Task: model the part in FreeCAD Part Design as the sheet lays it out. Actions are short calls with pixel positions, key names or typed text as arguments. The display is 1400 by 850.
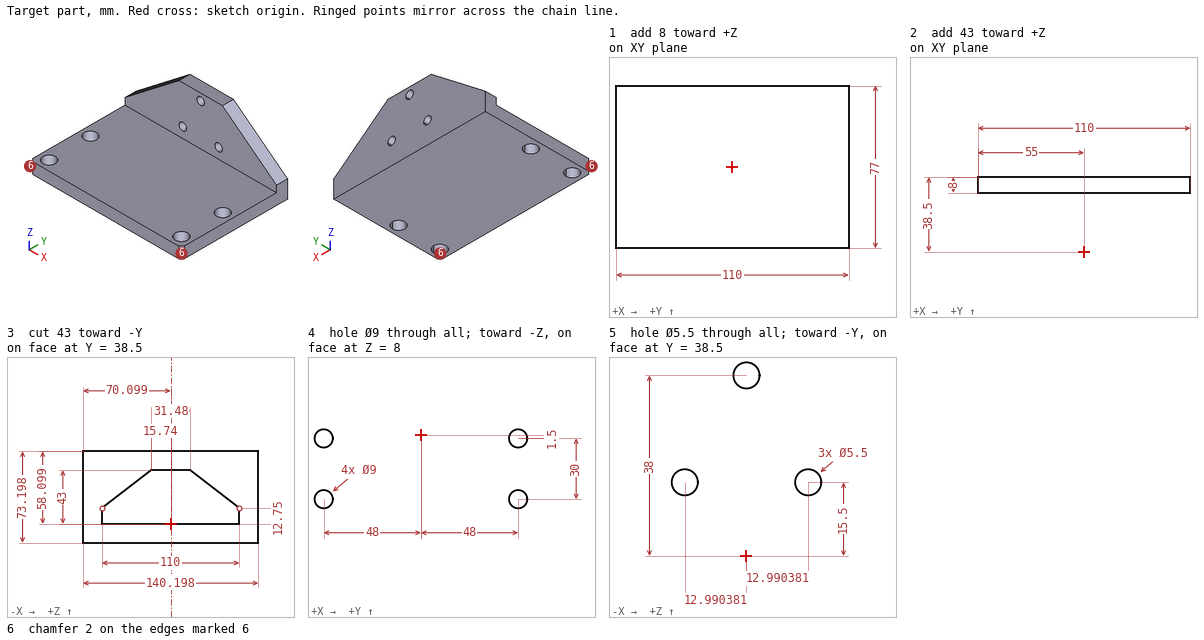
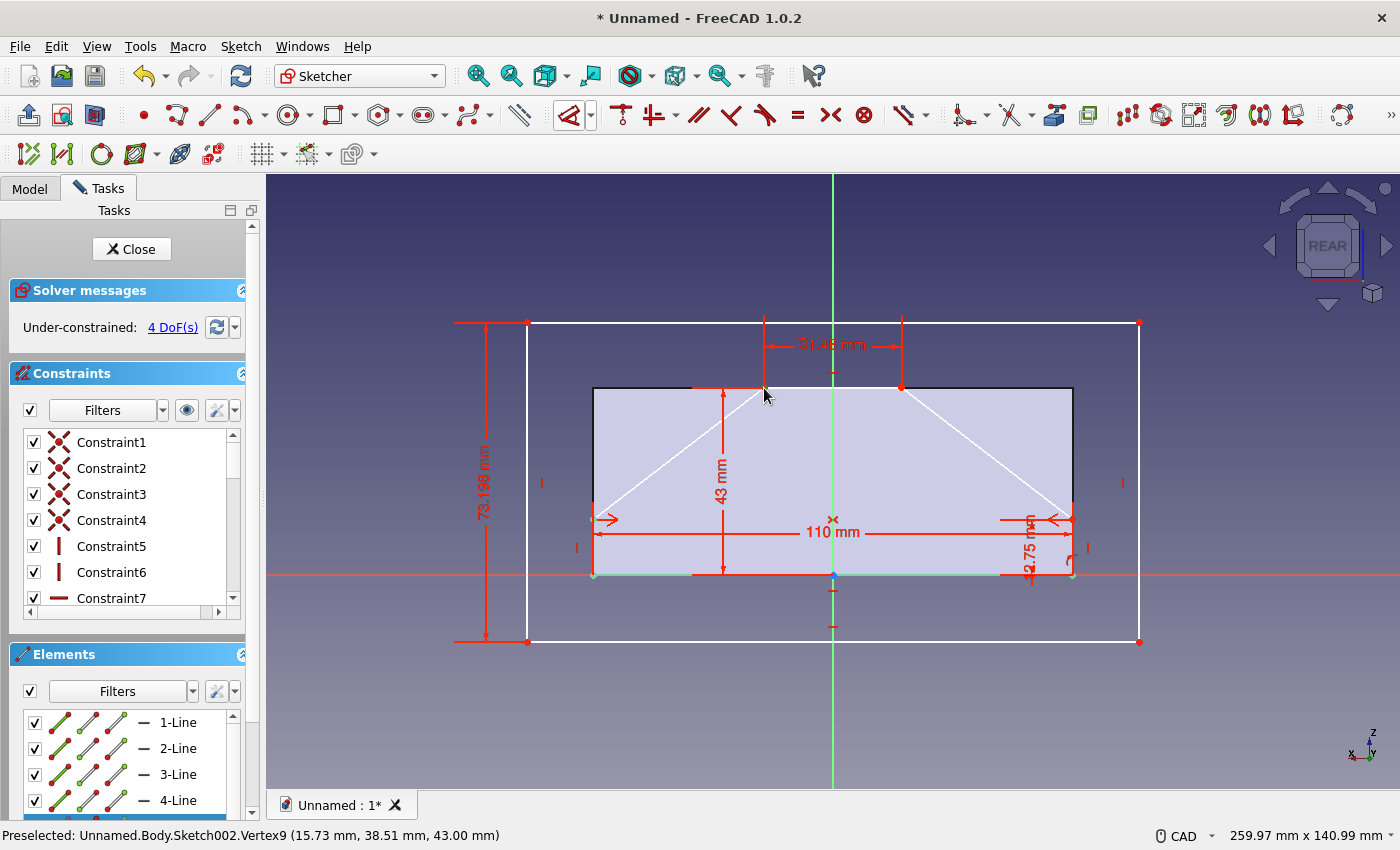
key(l)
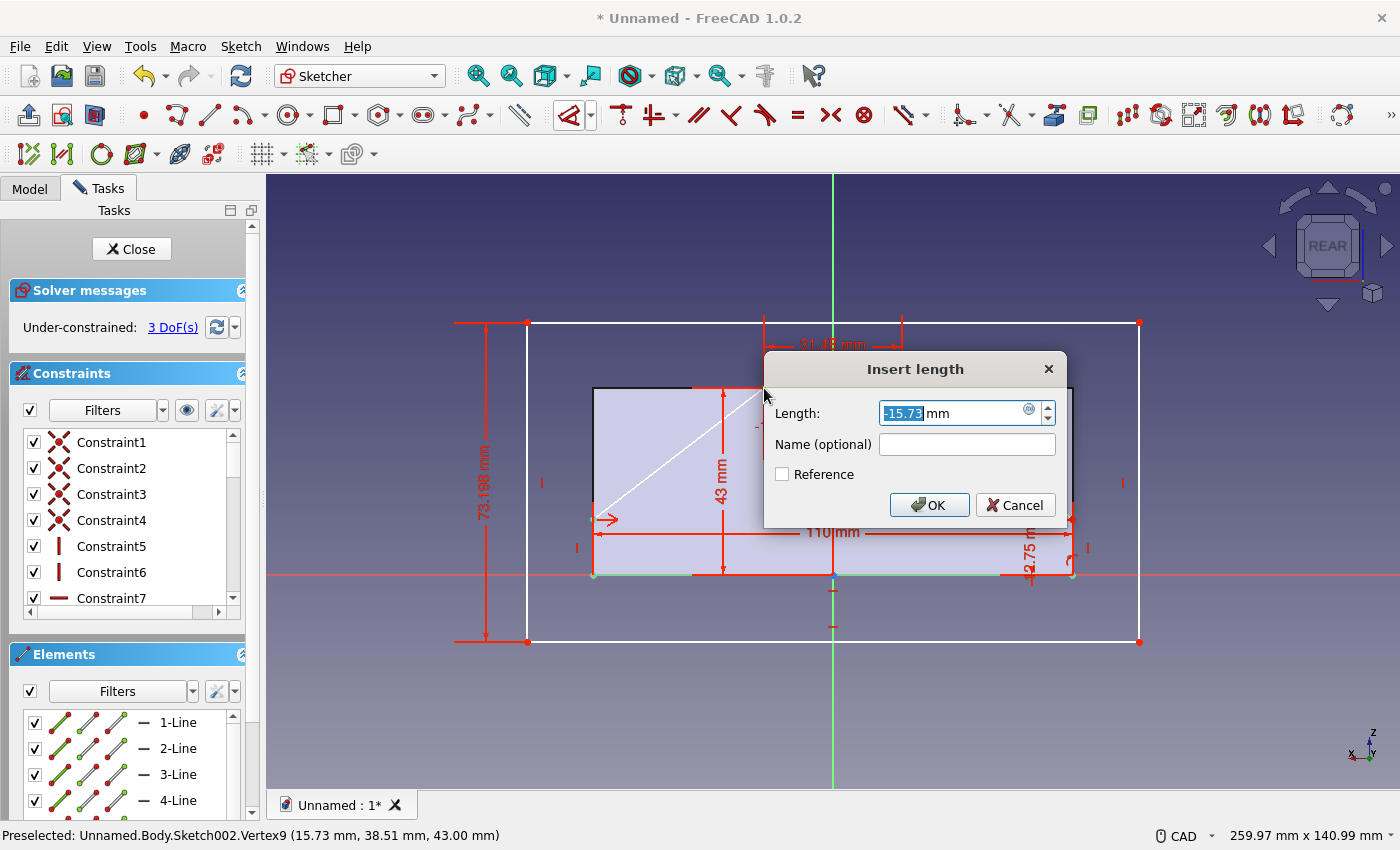
text(-15.74)
key(Return)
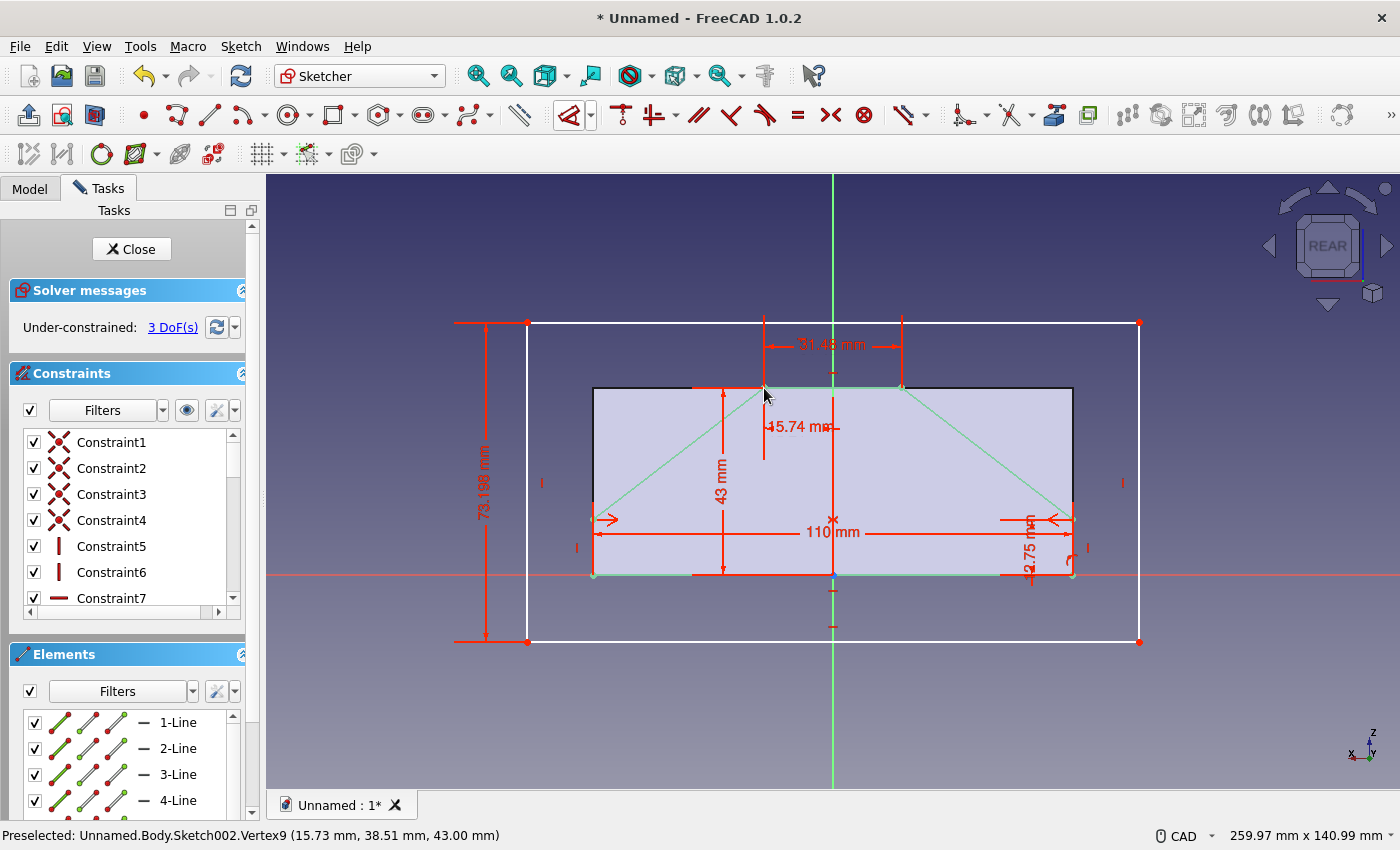
click(711, 642)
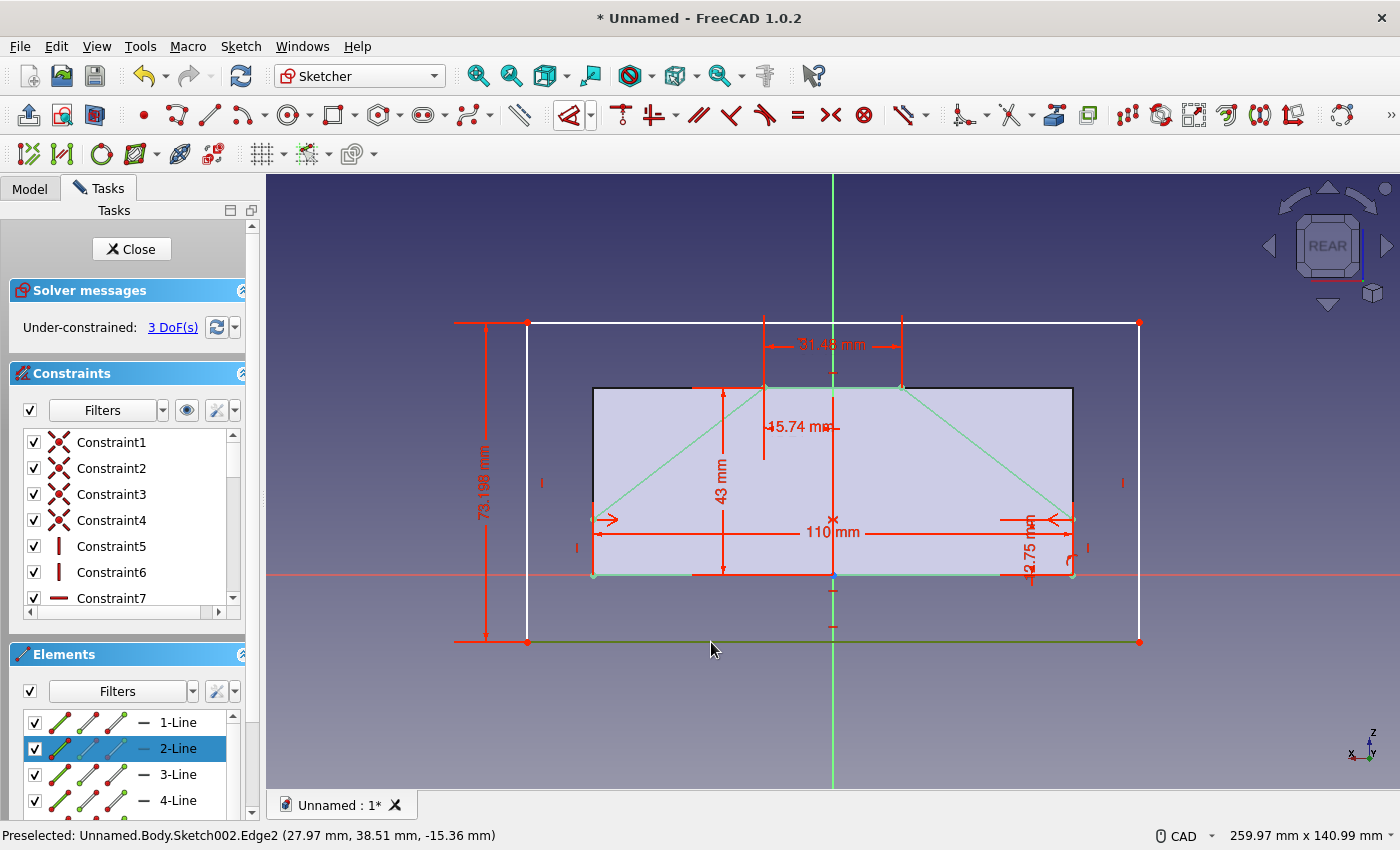
key(l)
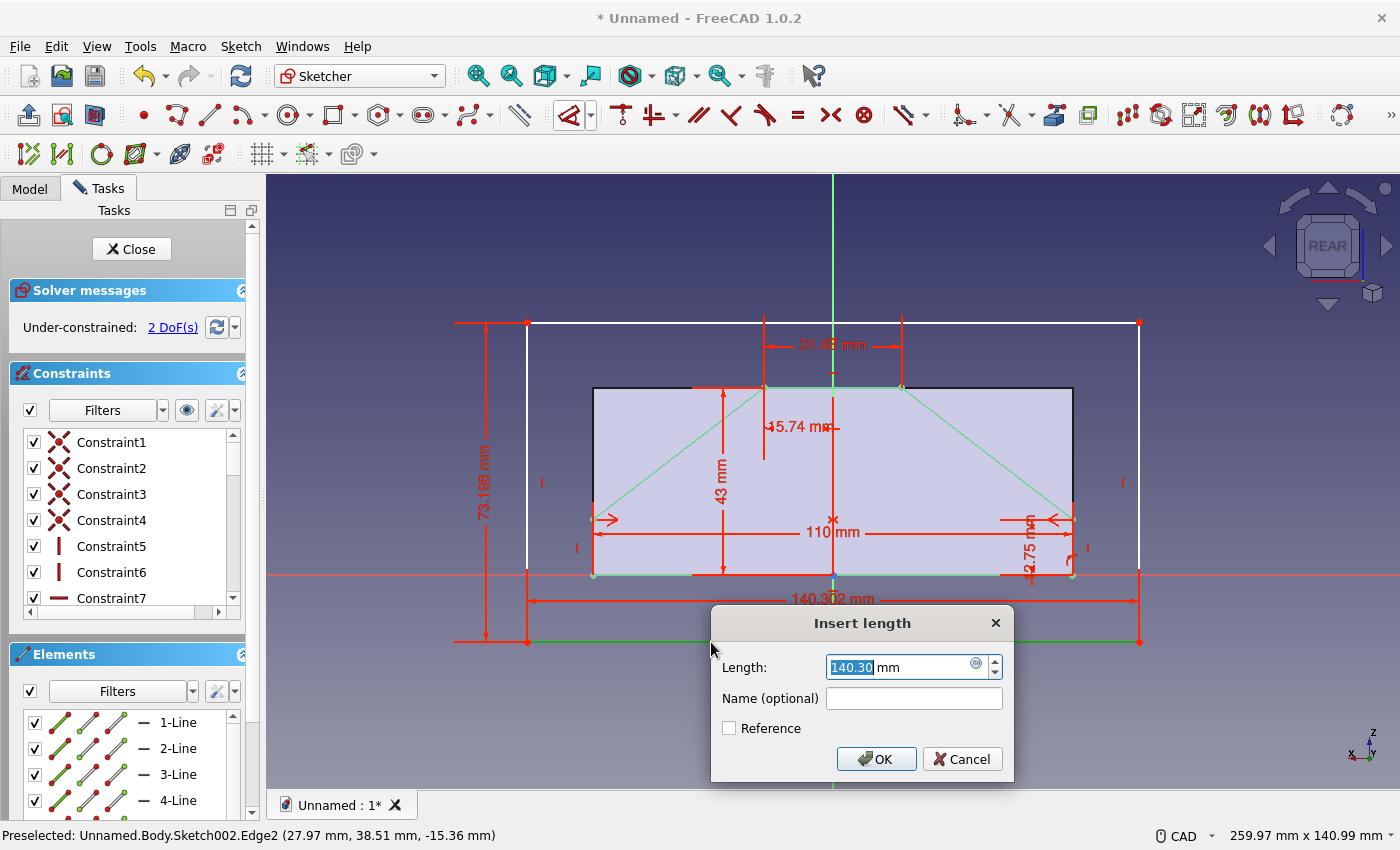
text(140.198)
key(Return)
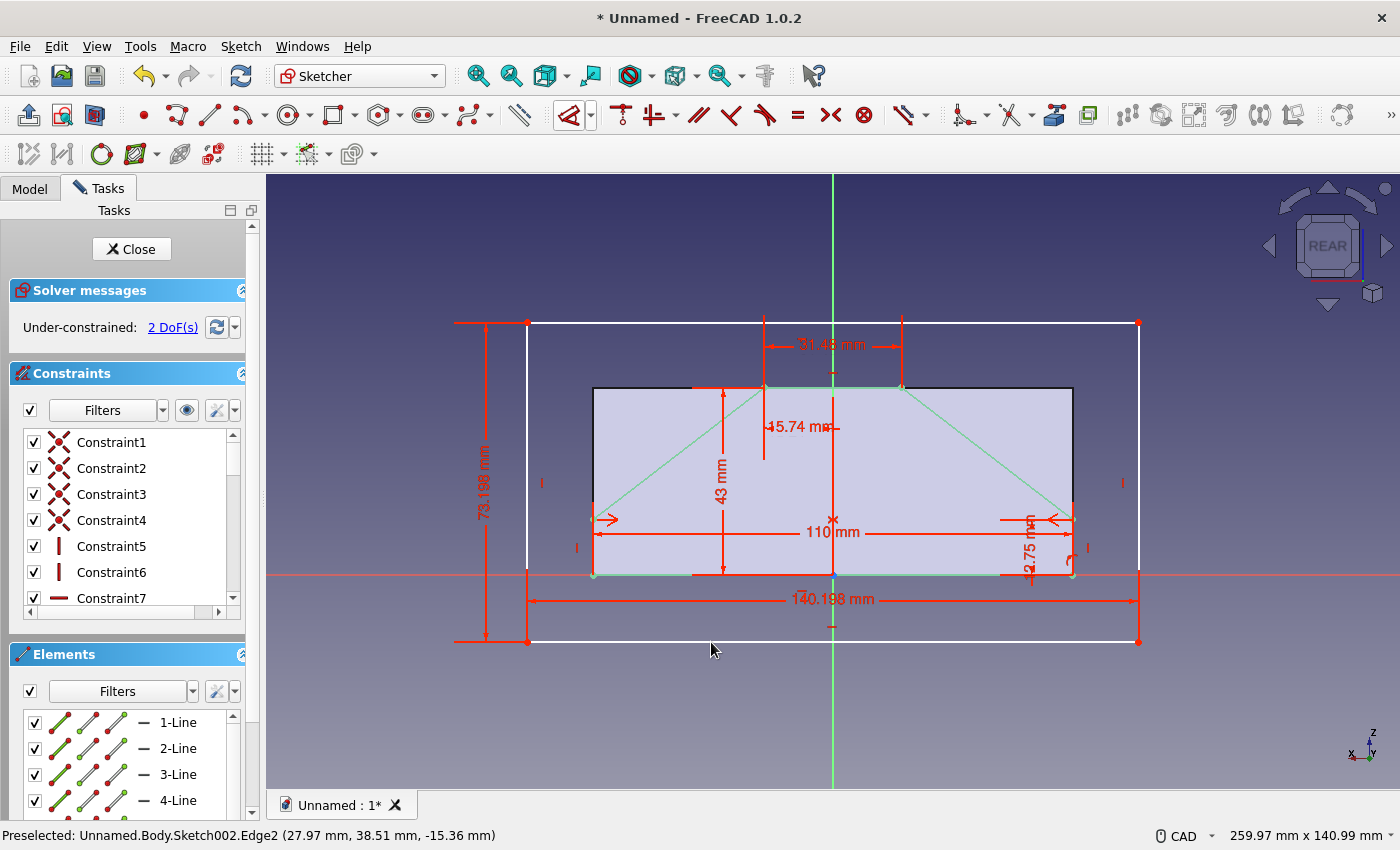
click(527, 323)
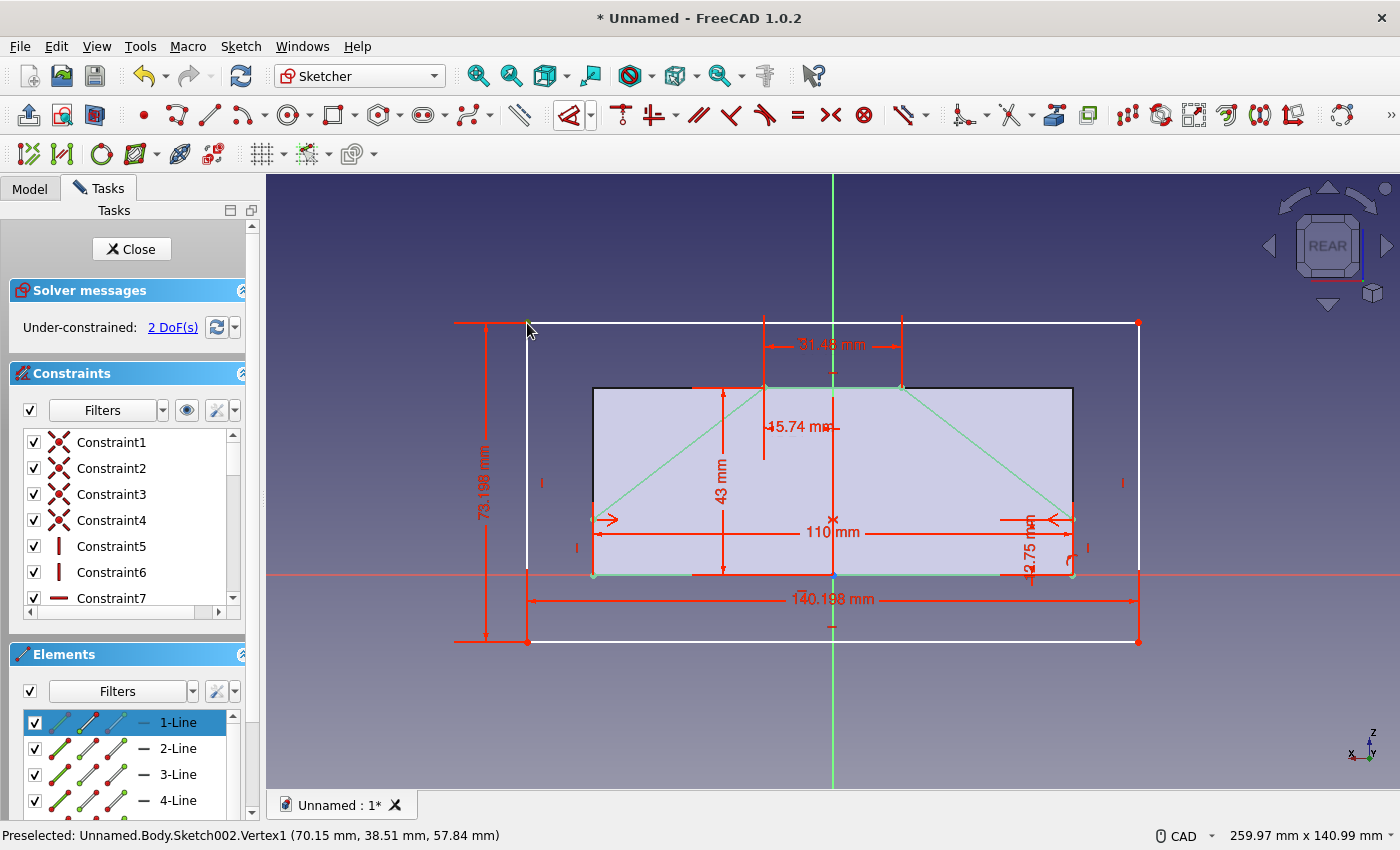
key(l)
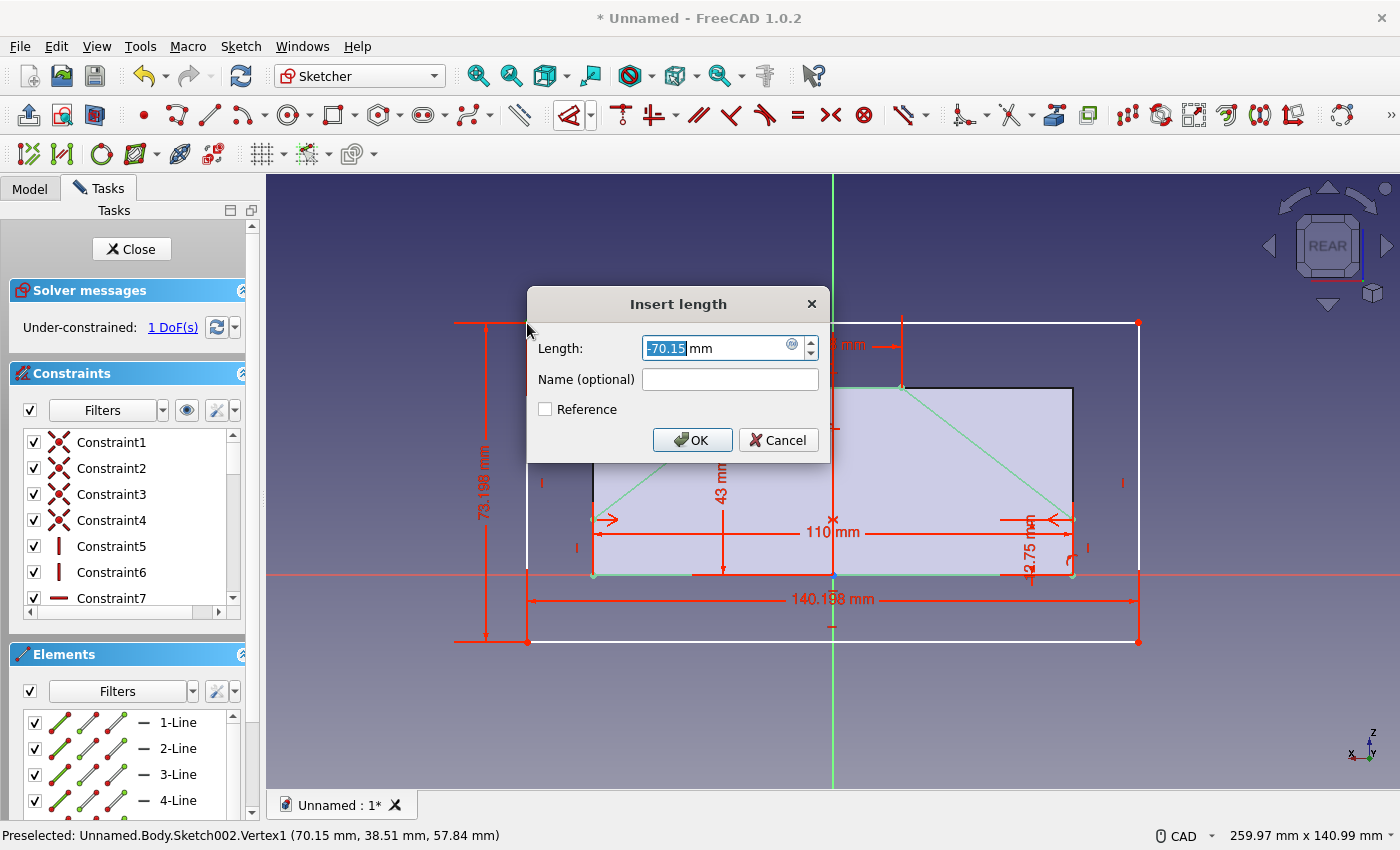
text(-70.099)
key(Return)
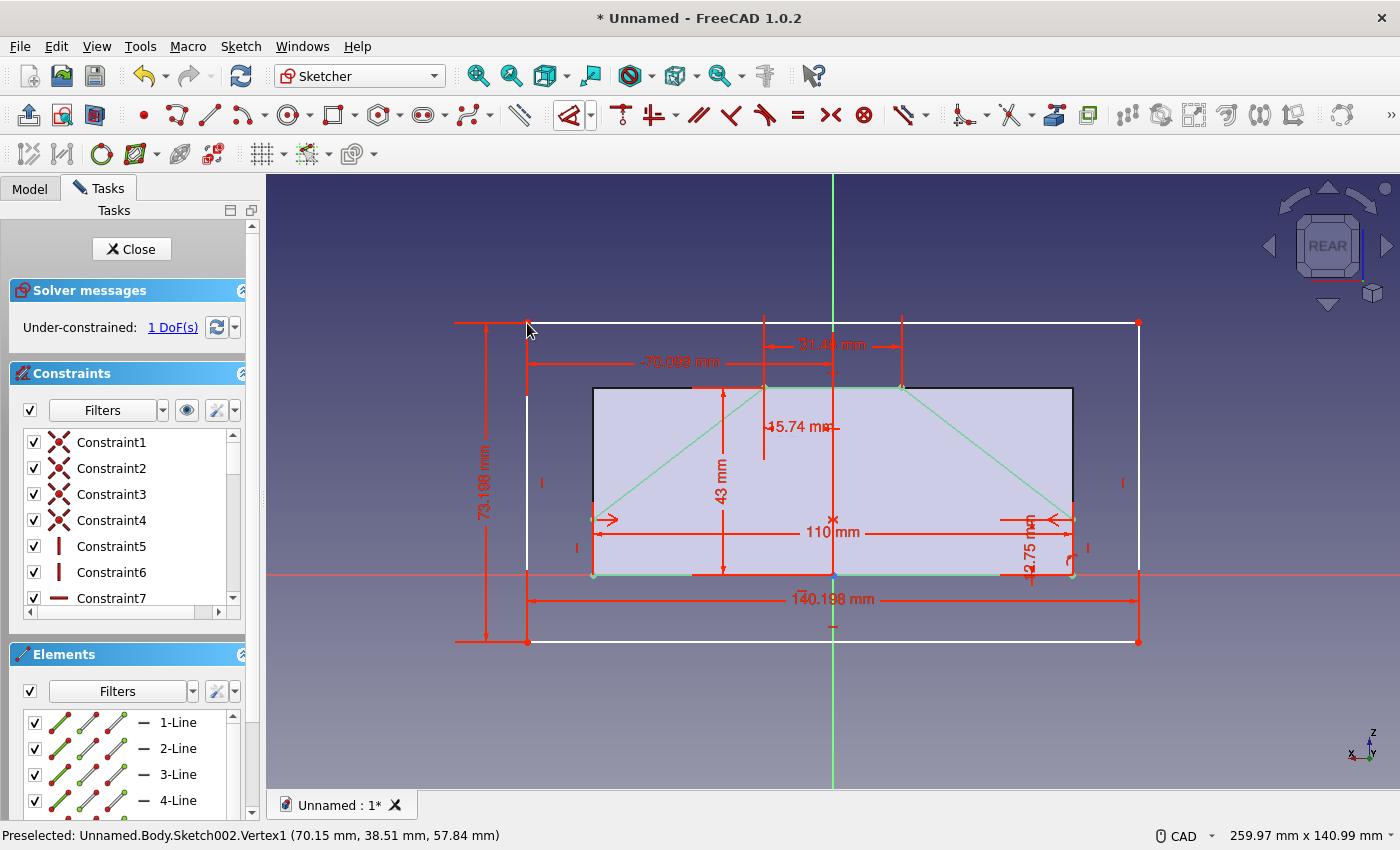
click(527, 323)